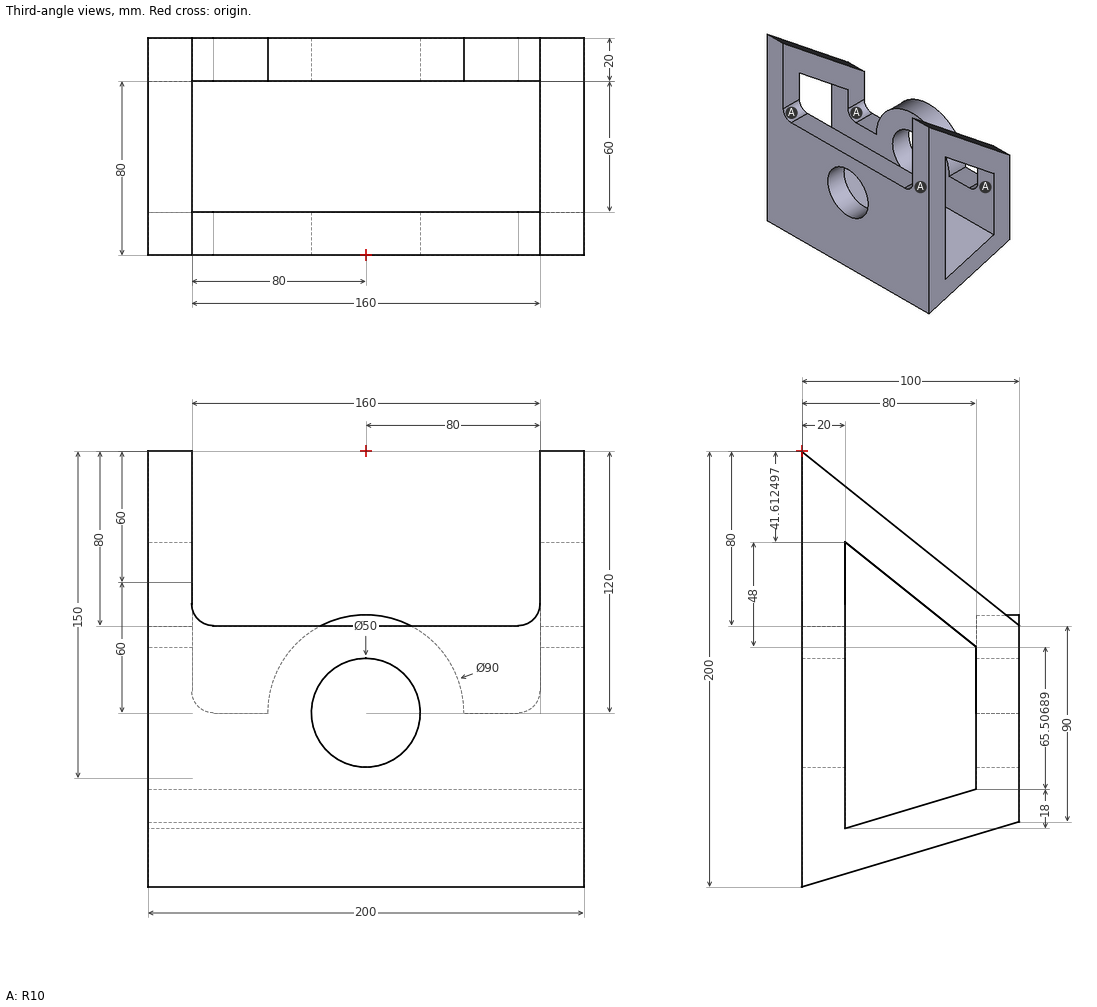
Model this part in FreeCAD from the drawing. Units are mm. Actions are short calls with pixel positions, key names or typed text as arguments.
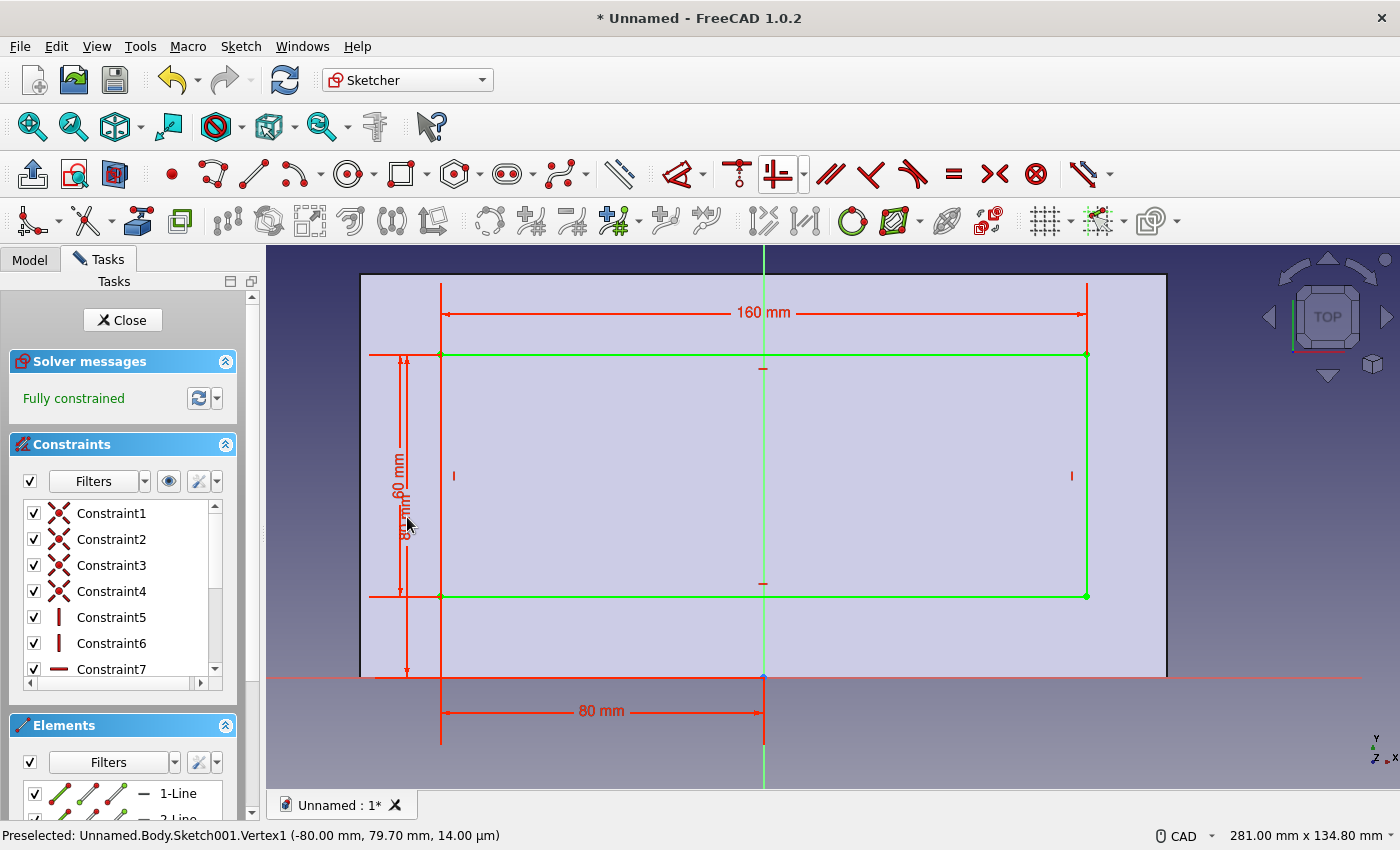
click(123, 320)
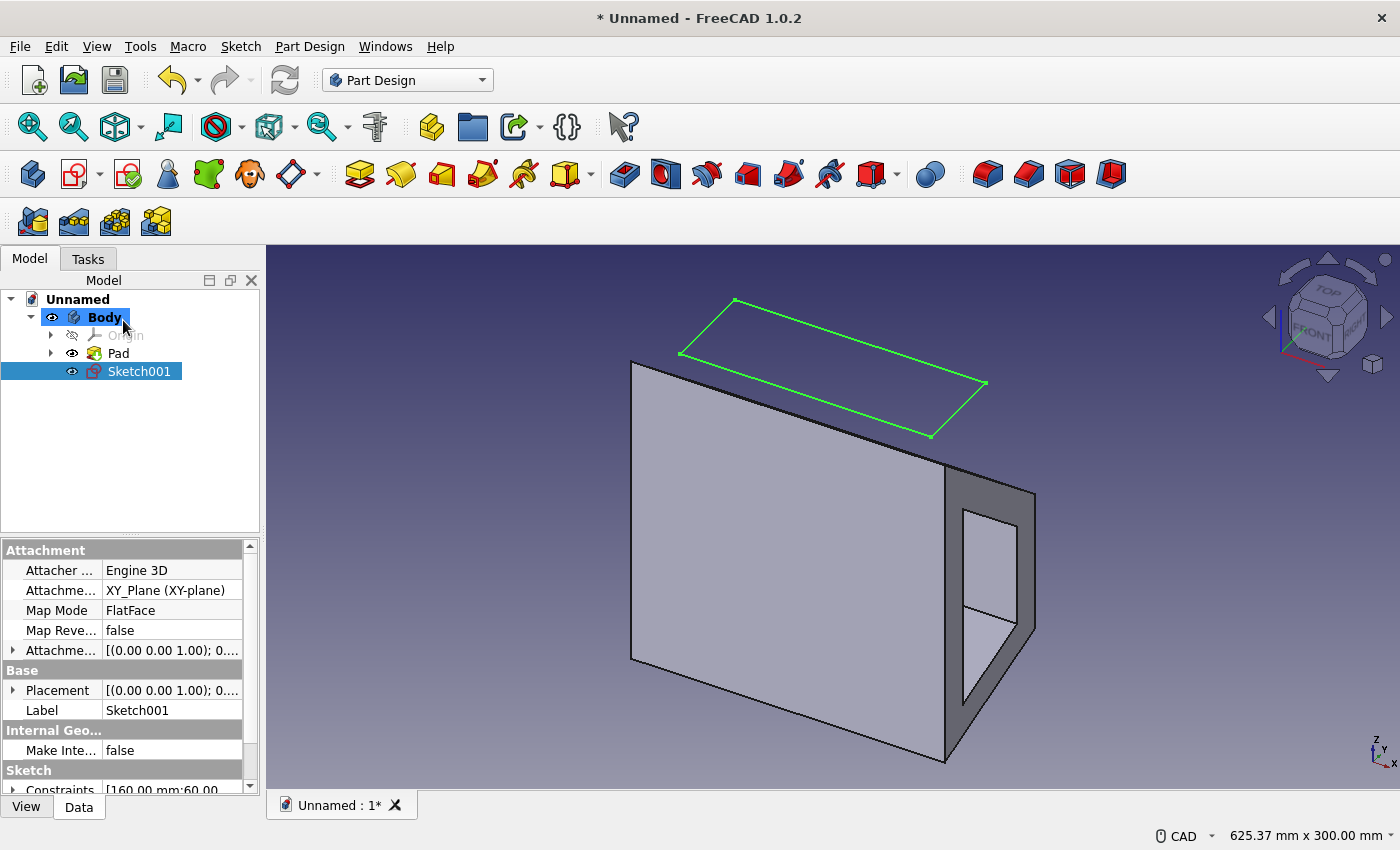
click(625, 174)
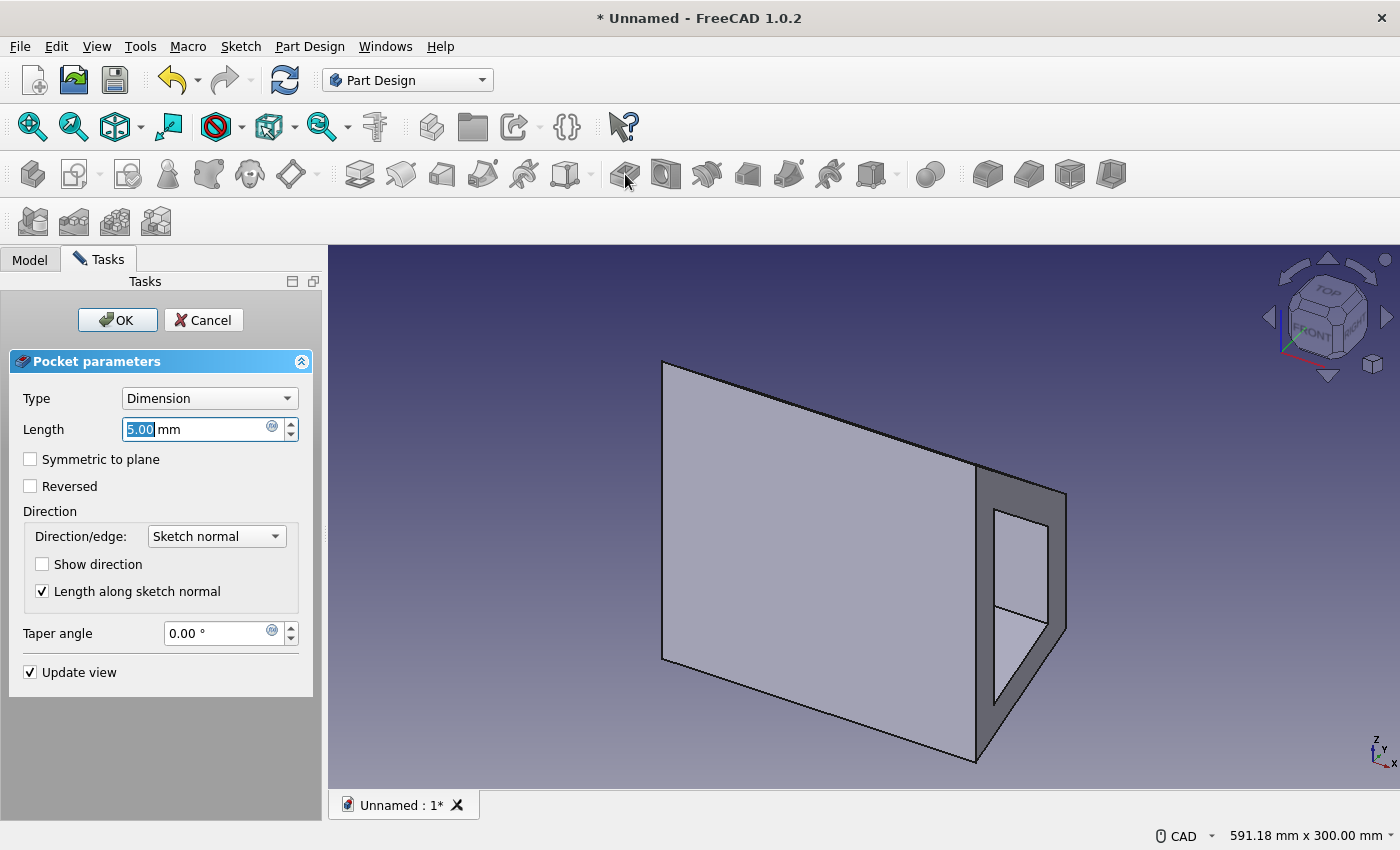
text(150)
key(Tab)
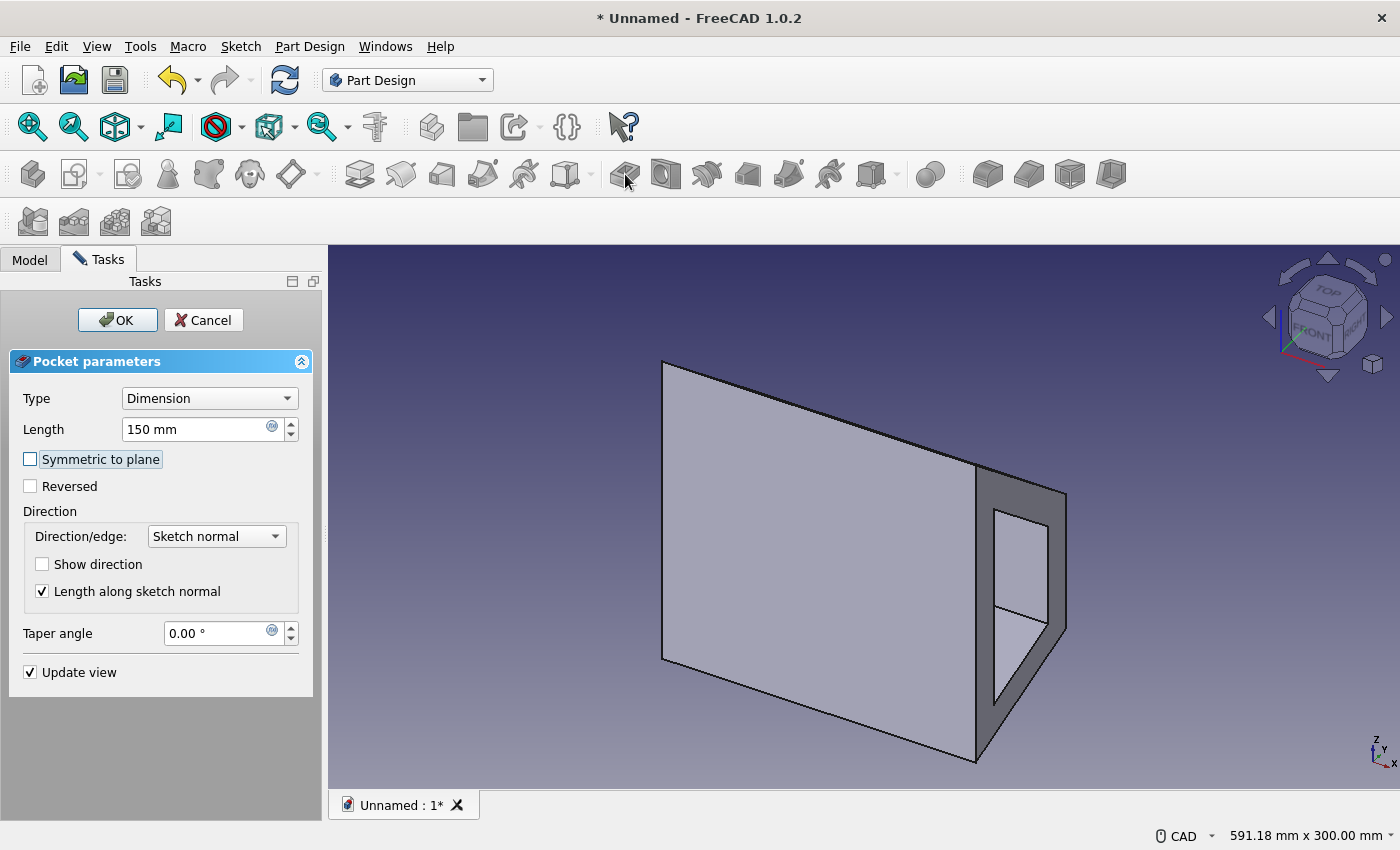
click(118, 320)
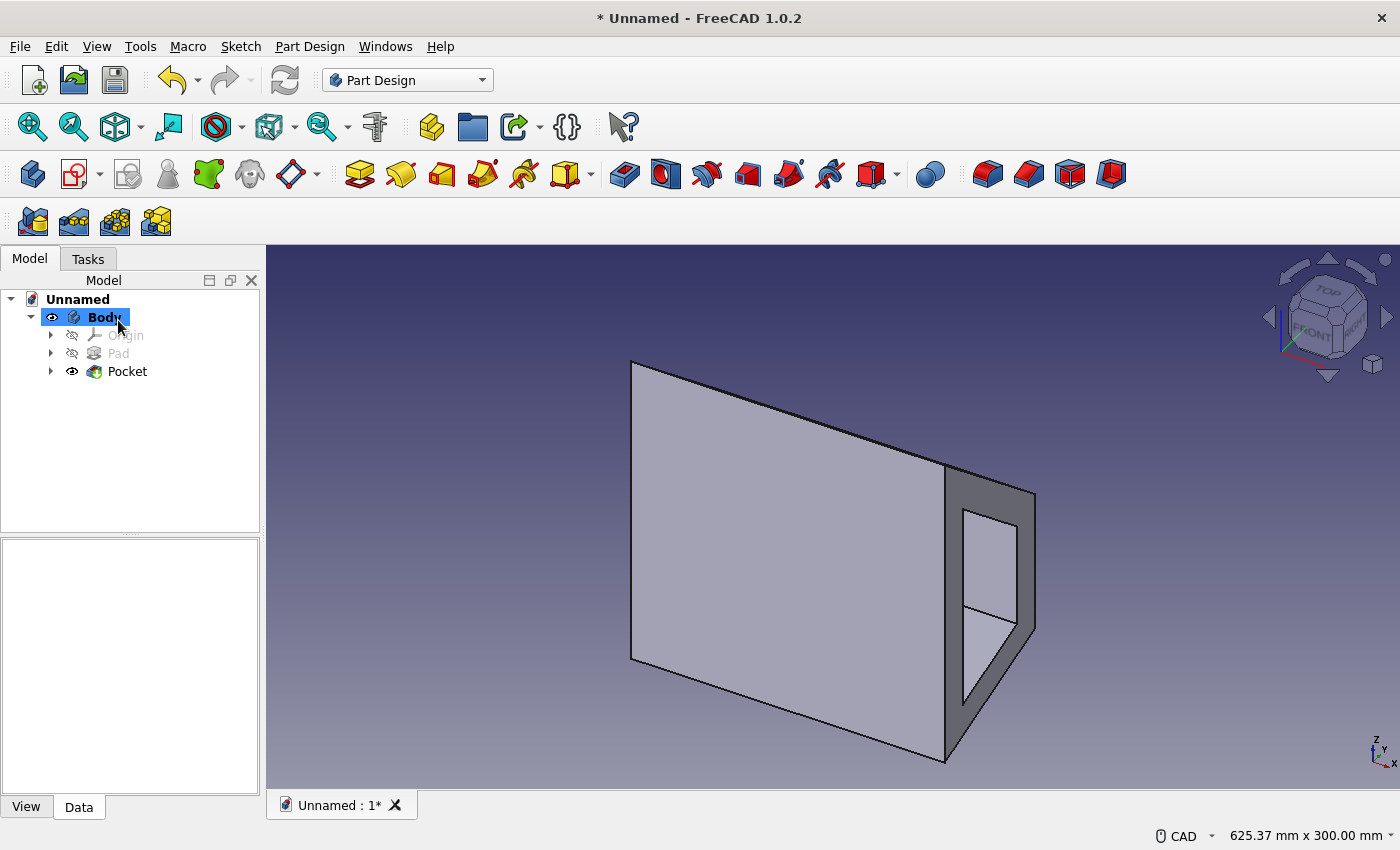
key(4)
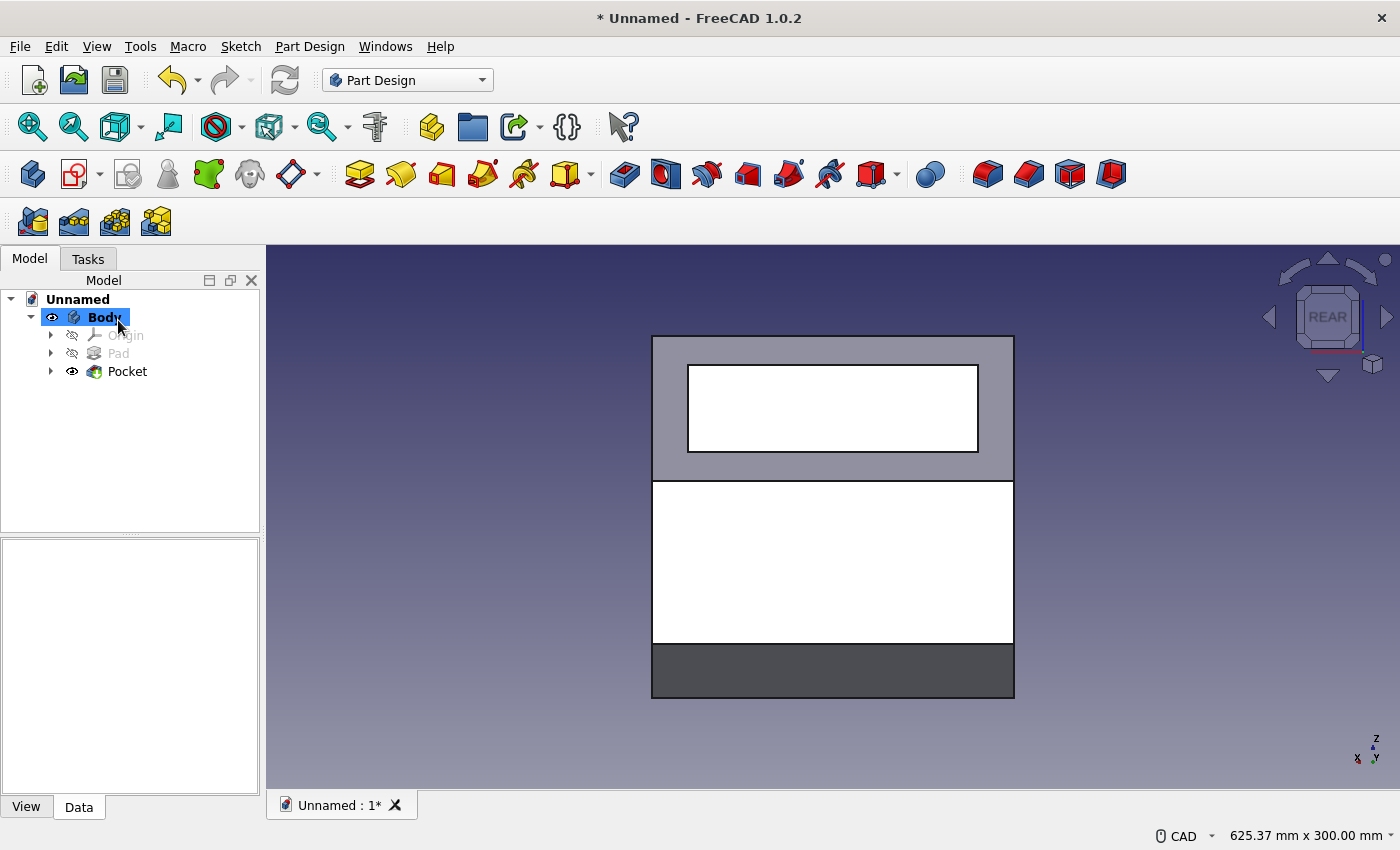
click(833, 561)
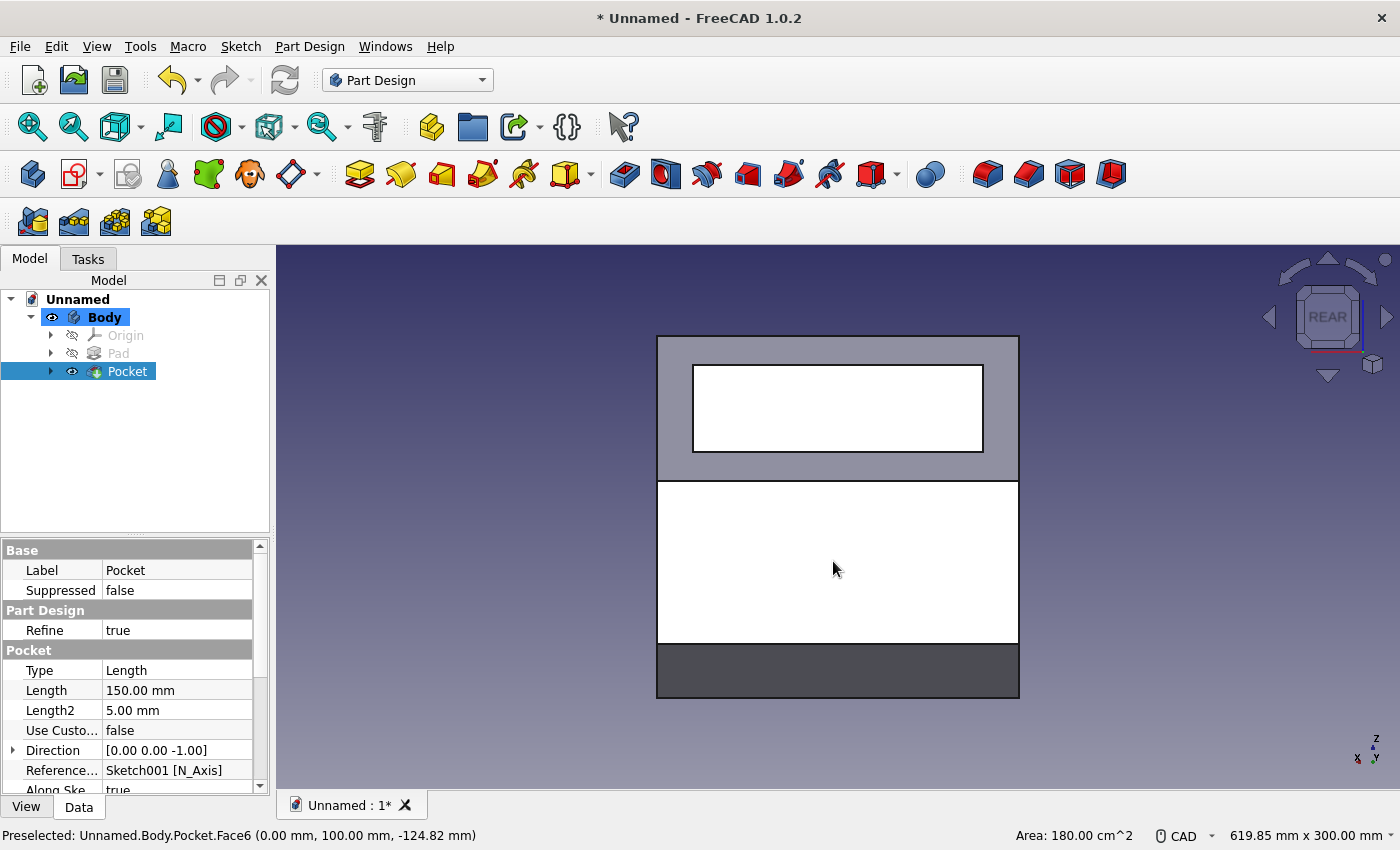
click(74, 174)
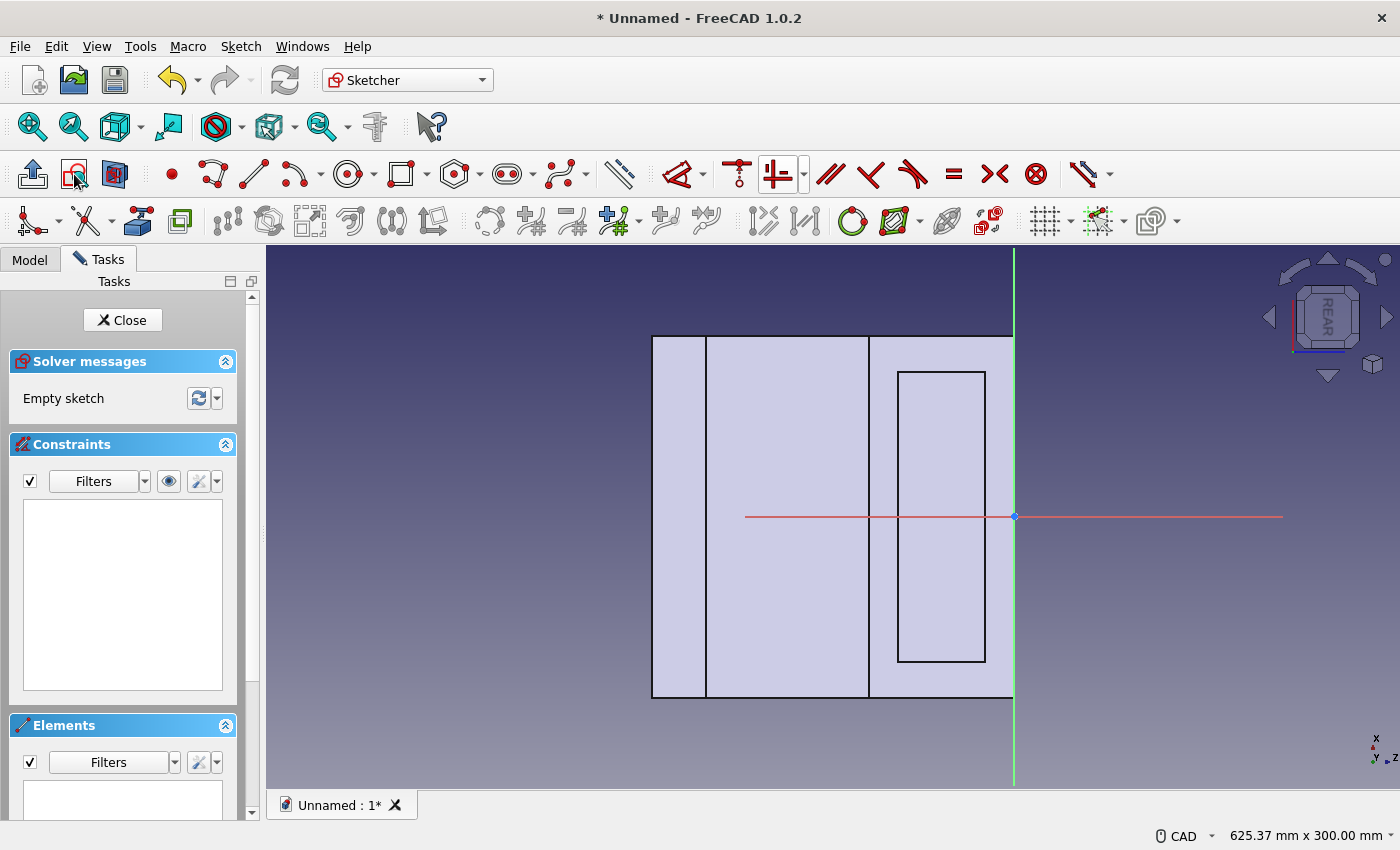
key(g)
key(r)